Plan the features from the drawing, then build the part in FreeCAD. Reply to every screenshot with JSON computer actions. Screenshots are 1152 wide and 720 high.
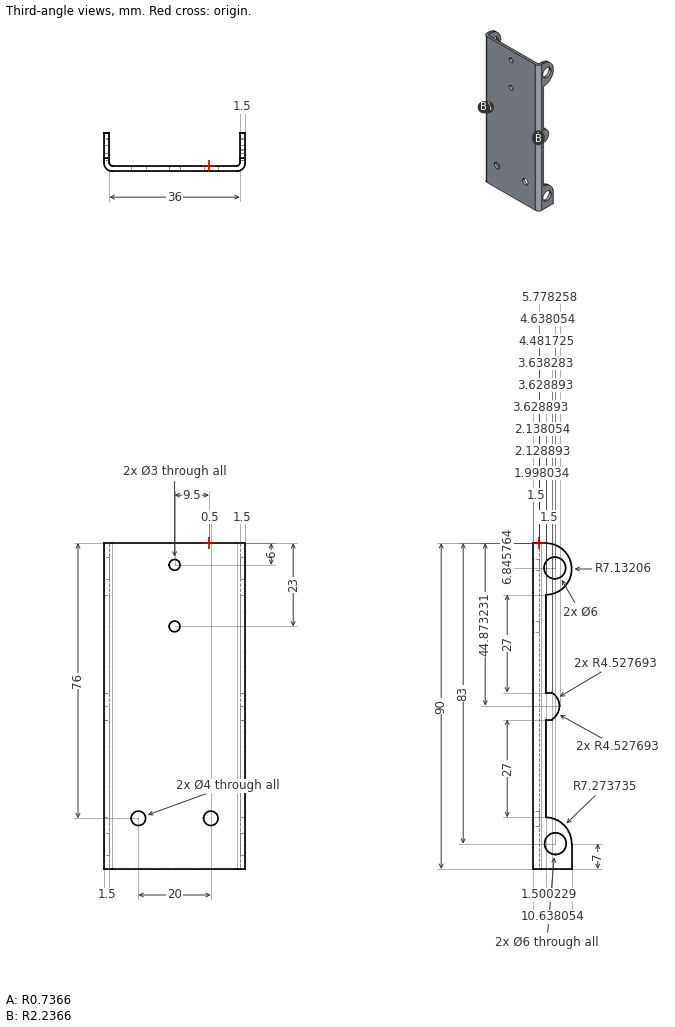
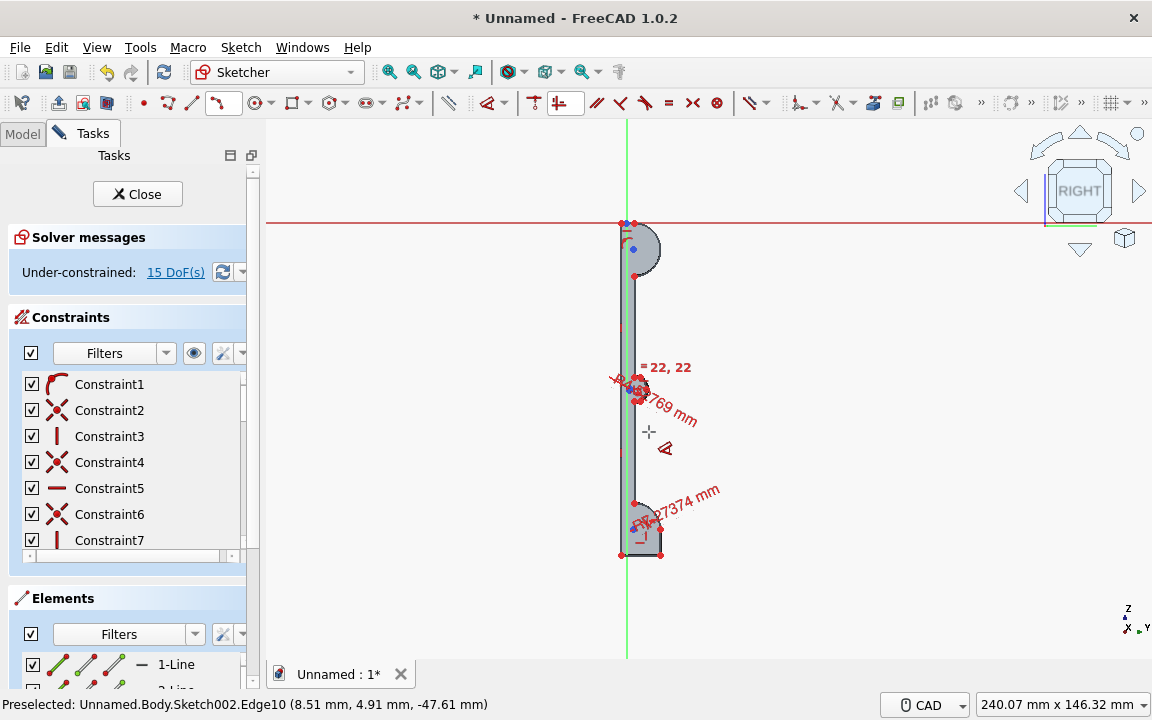
{"action": "scroll", "coordinate": [655, 265], "scroll_direction": "up", "scroll_amount": 3}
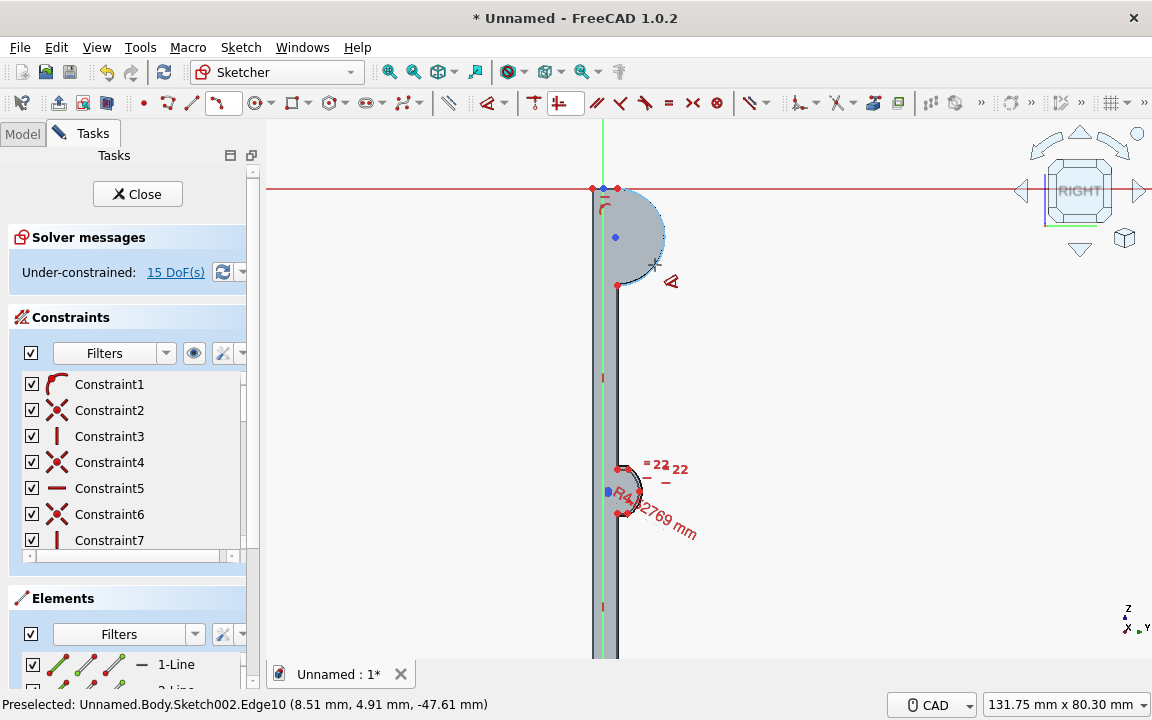
{"action": "left_click", "coordinate": [656, 265]}
{"action": "left_click", "coordinate": [682, 283]}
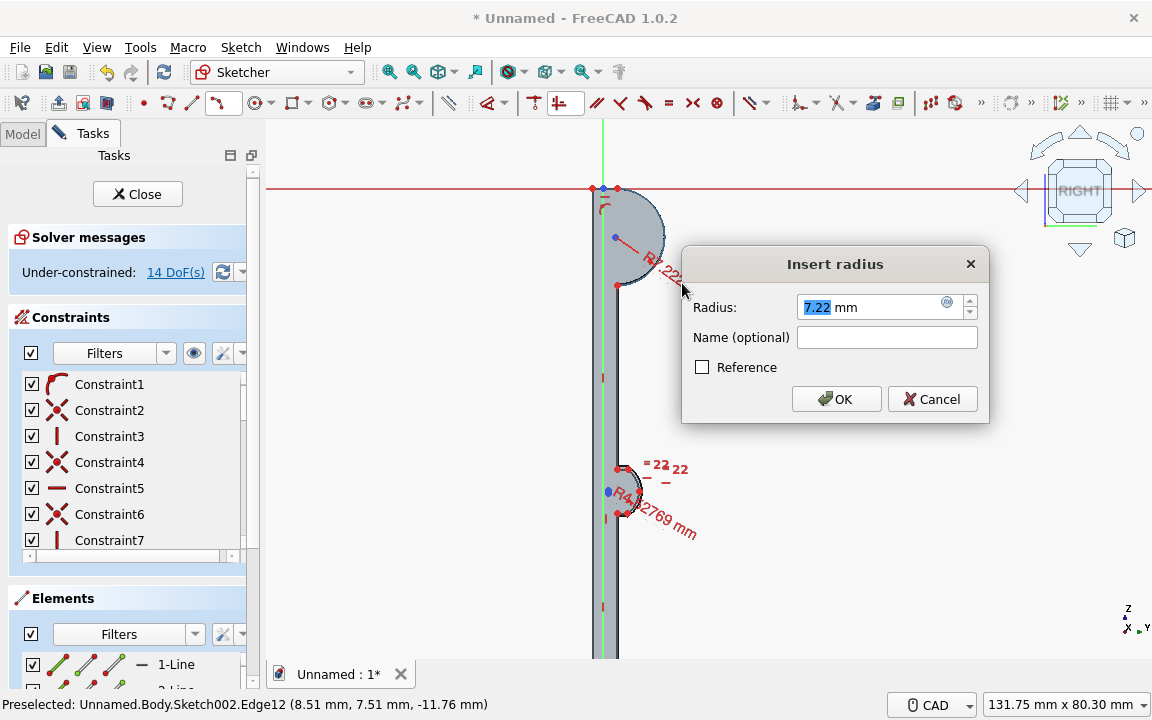
{"action": "type", "text": "7.13206"}
{"action": "key", "text": "Return"}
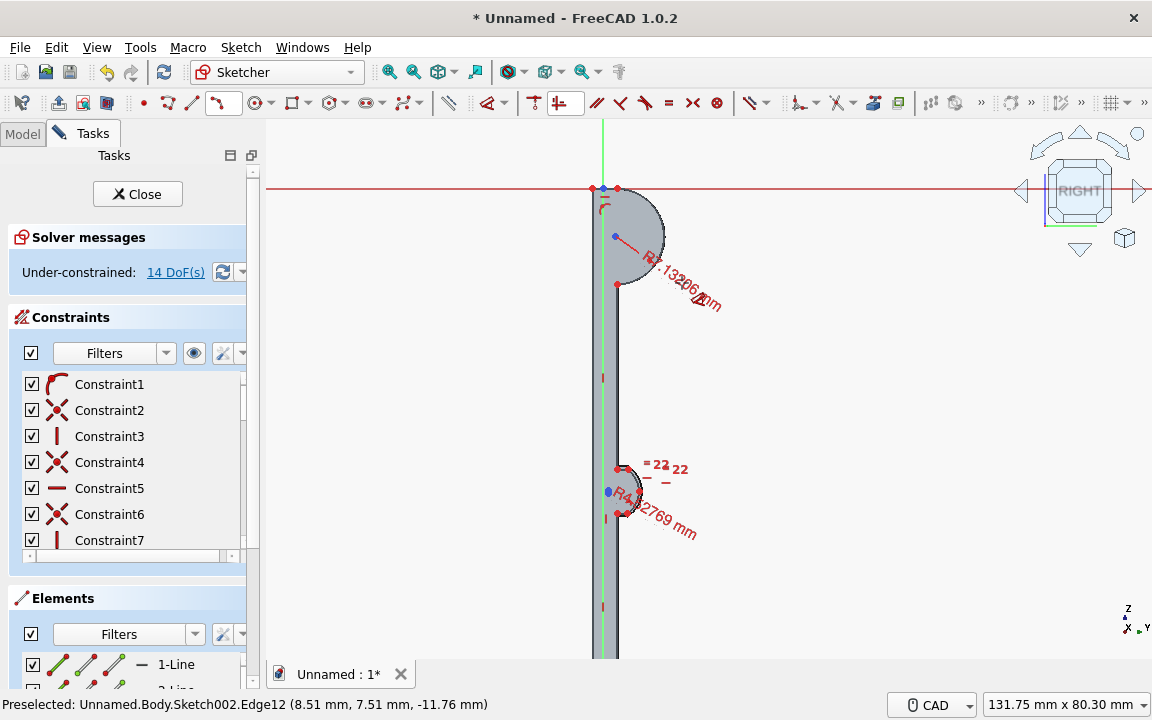
{"action": "scroll", "coordinate": [655, 265], "scroll_direction": "down", "scroll_amount": 3}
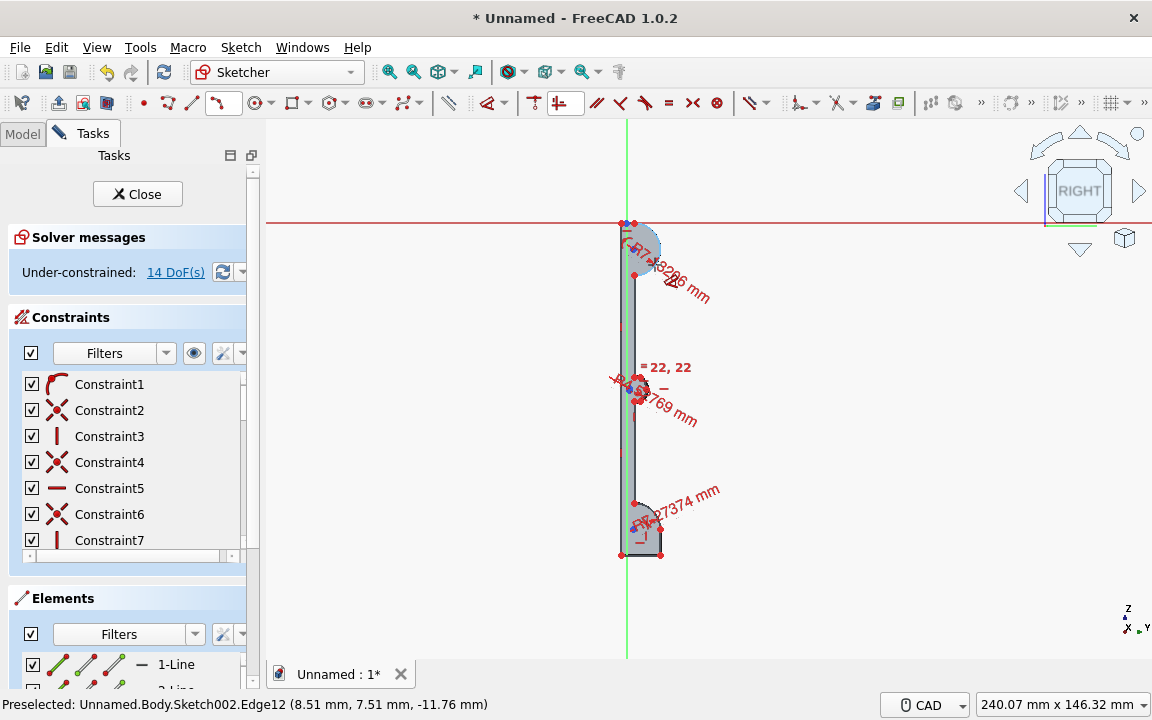
{"action": "scroll", "coordinate": [660, 548], "scroll_direction": "up", "scroll_amount": 3}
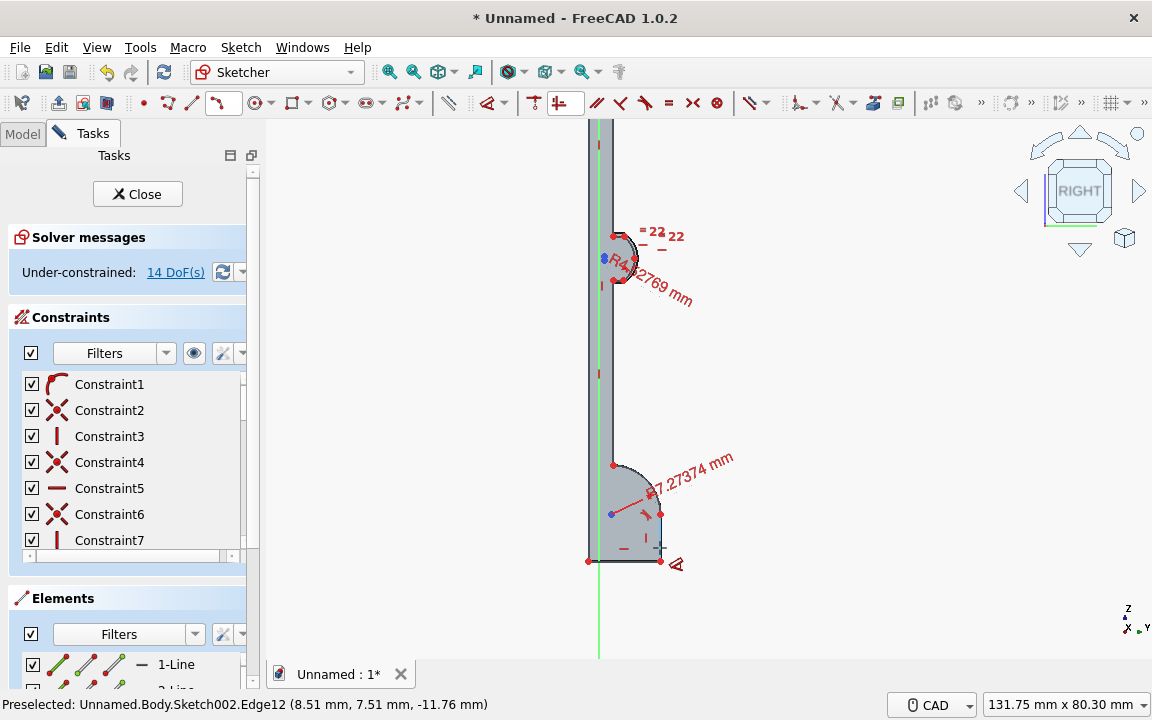
{"action": "left_click", "coordinate": [660, 547]}
{"action": "left_click", "coordinate": [694, 538]}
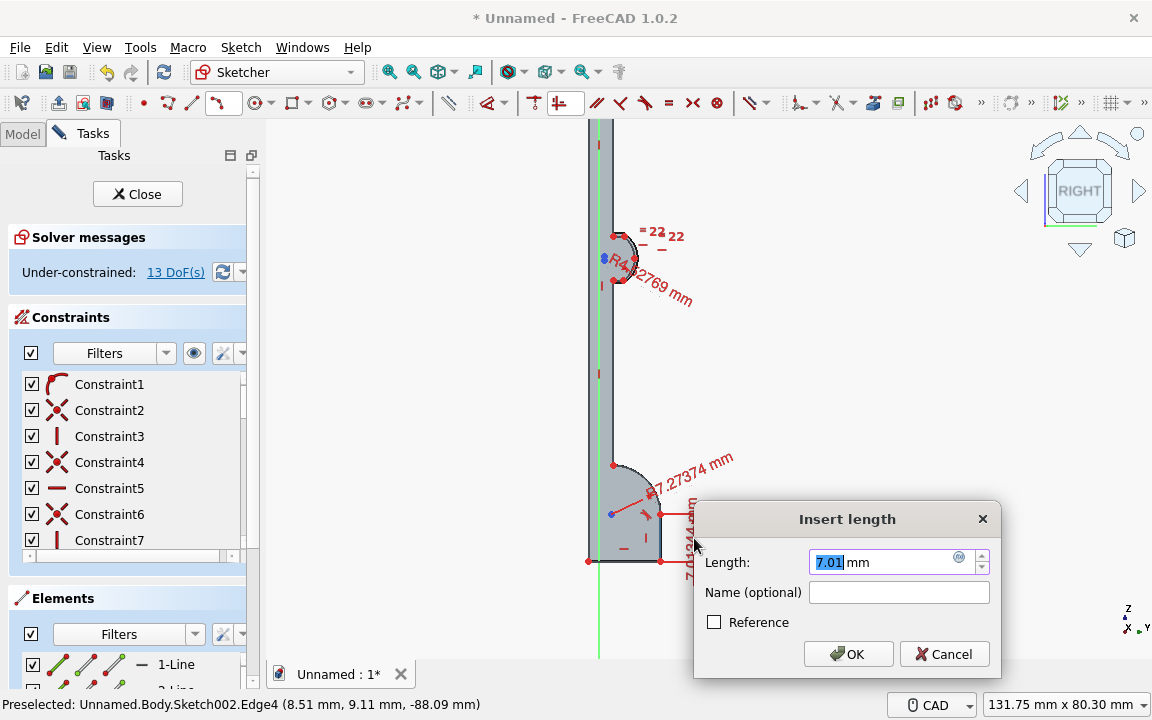
{"action": "type", "text": "7"}
{"action": "key", "text": "Return"}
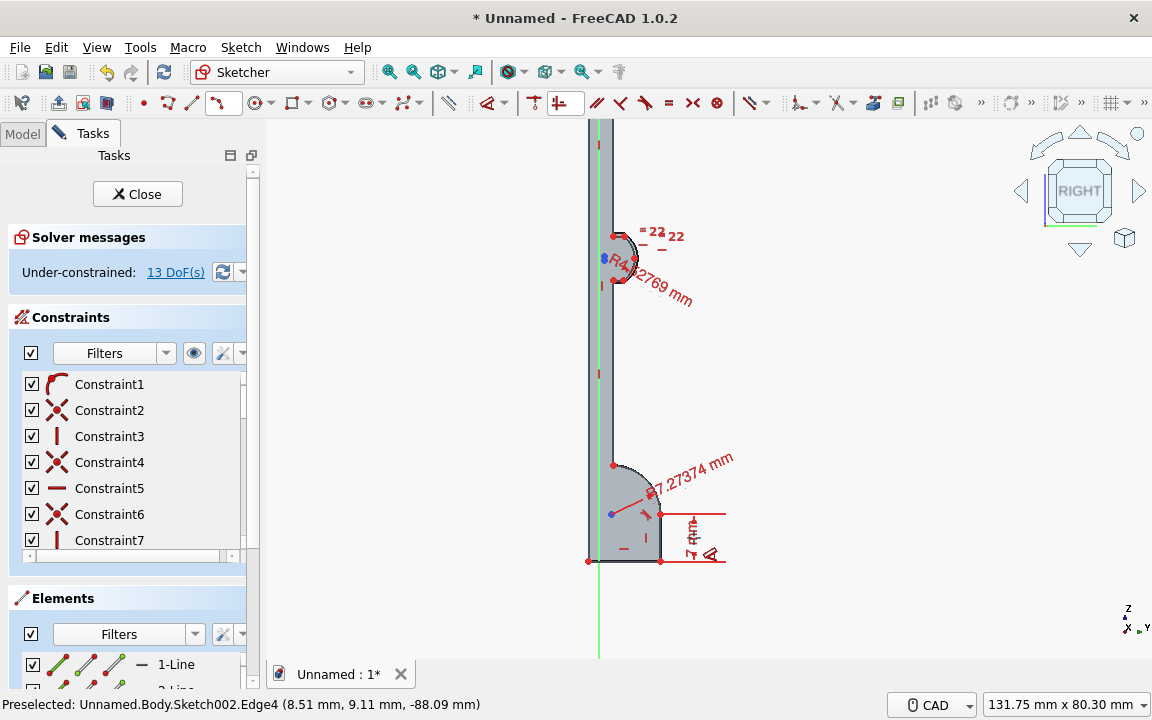
{"action": "scroll", "coordinate": [589, 380], "scroll_direction": "up", "scroll_amount": 2}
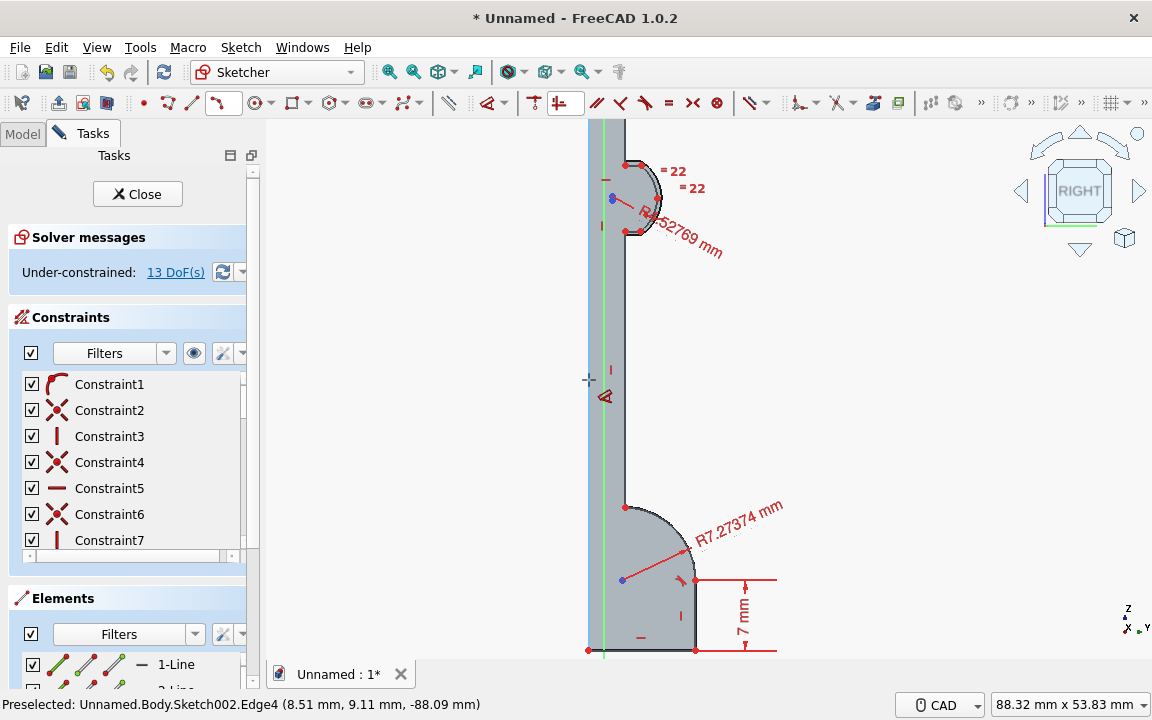
{"action": "left_click", "coordinate": [589, 379]}
{"action": "left_click", "coordinate": [555, 389]}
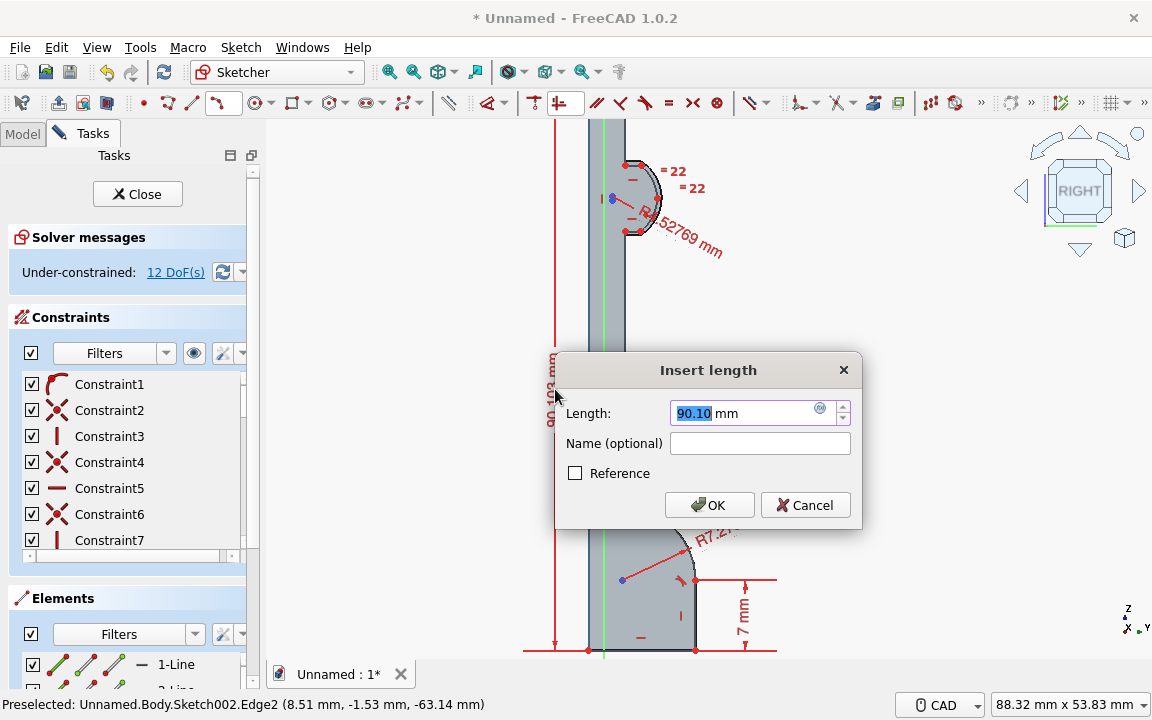
{"action": "type", "text": "90"}
{"action": "key", "text": "Return"}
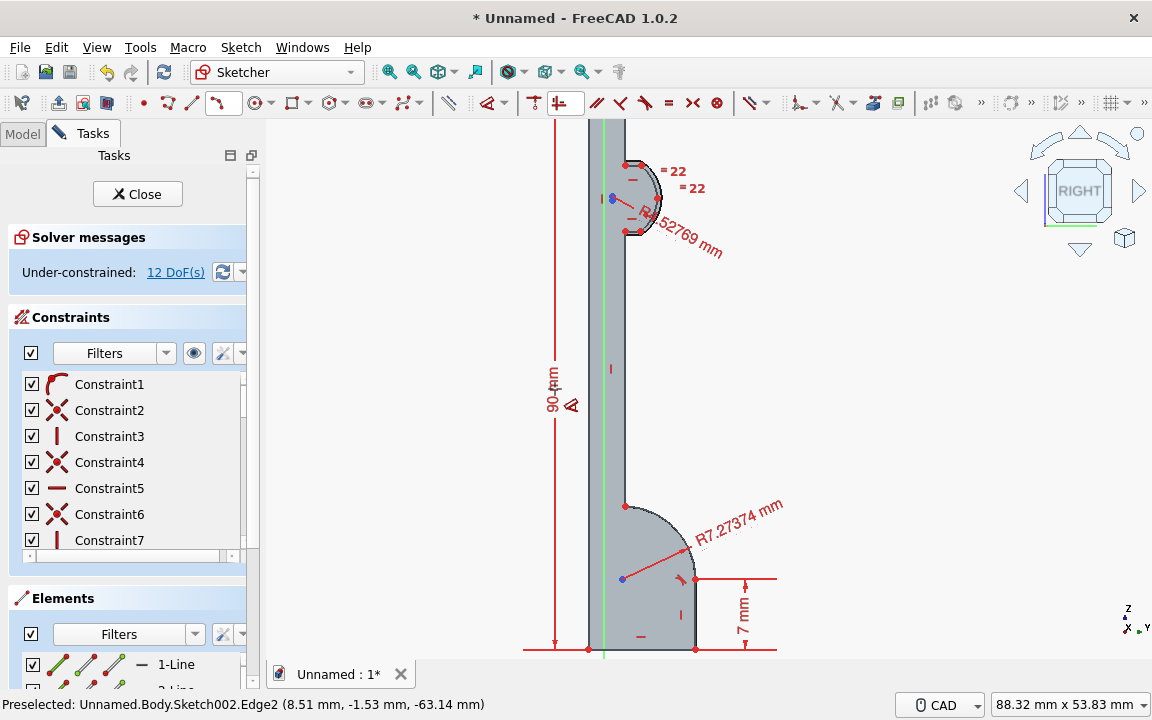
{"action": "left_click", "coordinate": [625, 424]}
{"action": "left_click", "coordinate": [659, 369]}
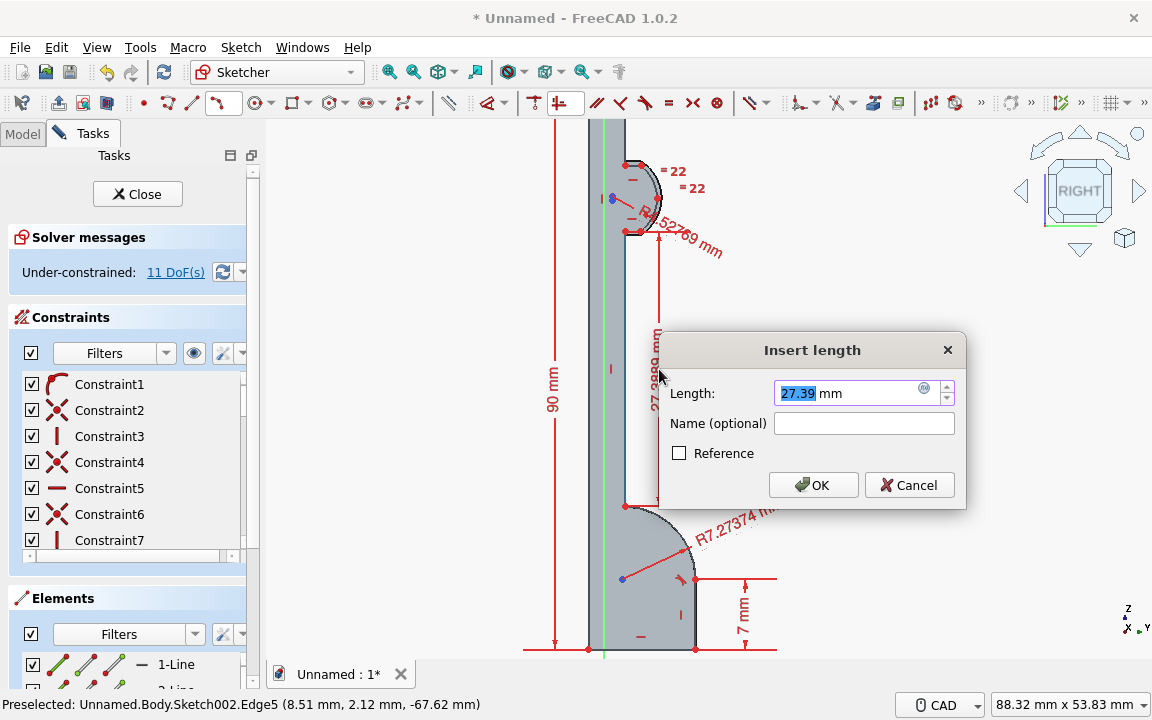
{"action": "type", "text": "27"}
{"action": "key", "text": "Return"}